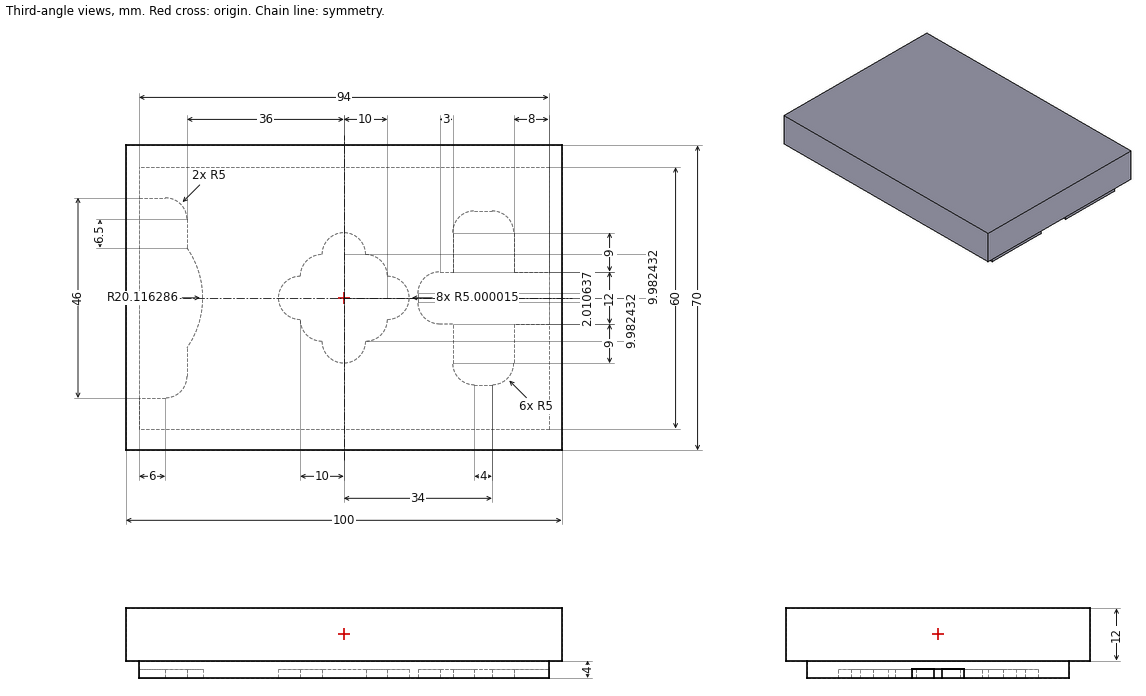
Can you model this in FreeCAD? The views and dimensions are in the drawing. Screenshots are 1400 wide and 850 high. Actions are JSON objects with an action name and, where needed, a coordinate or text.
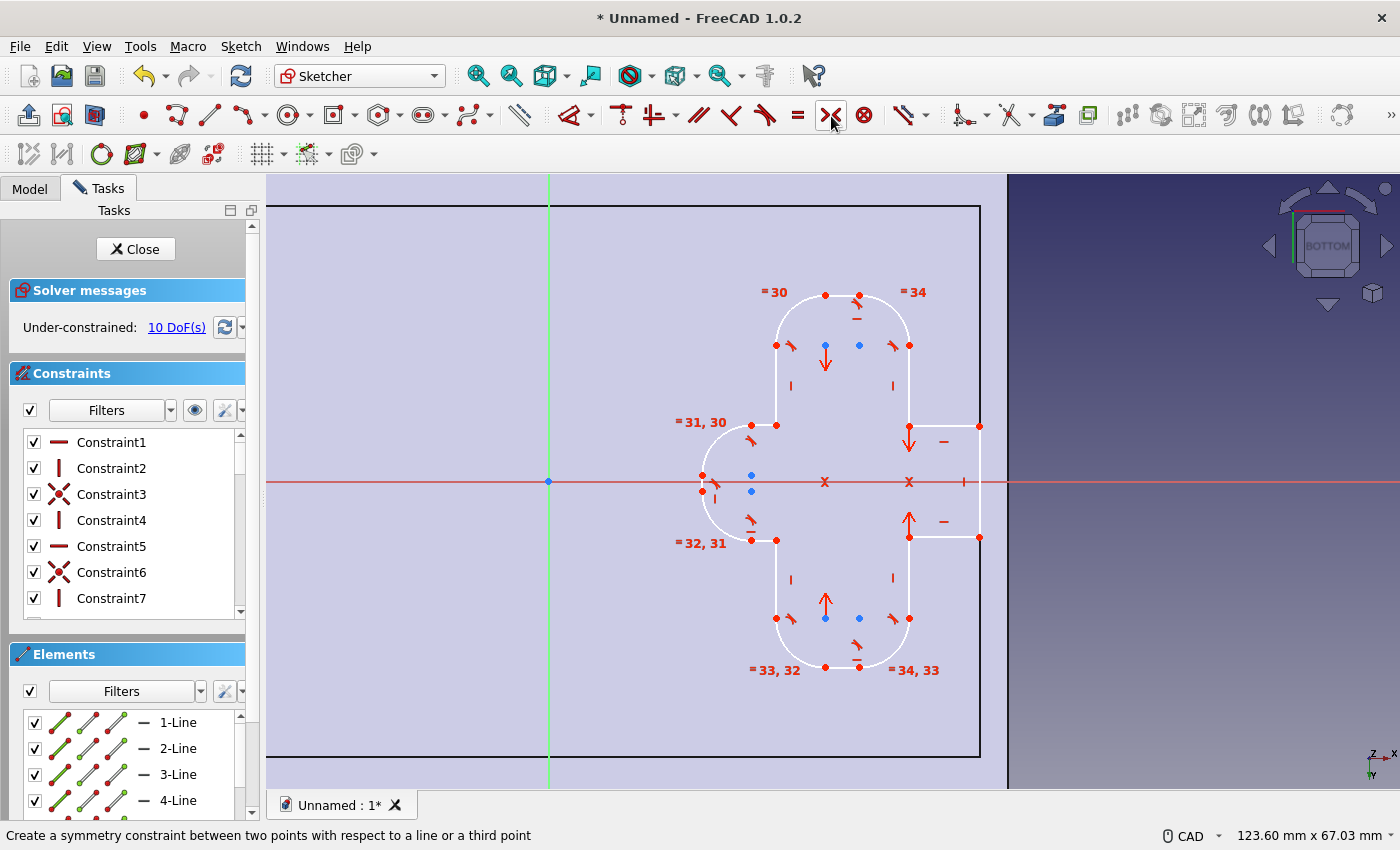
{"action": "left_click", "coordinate": [568, 116]}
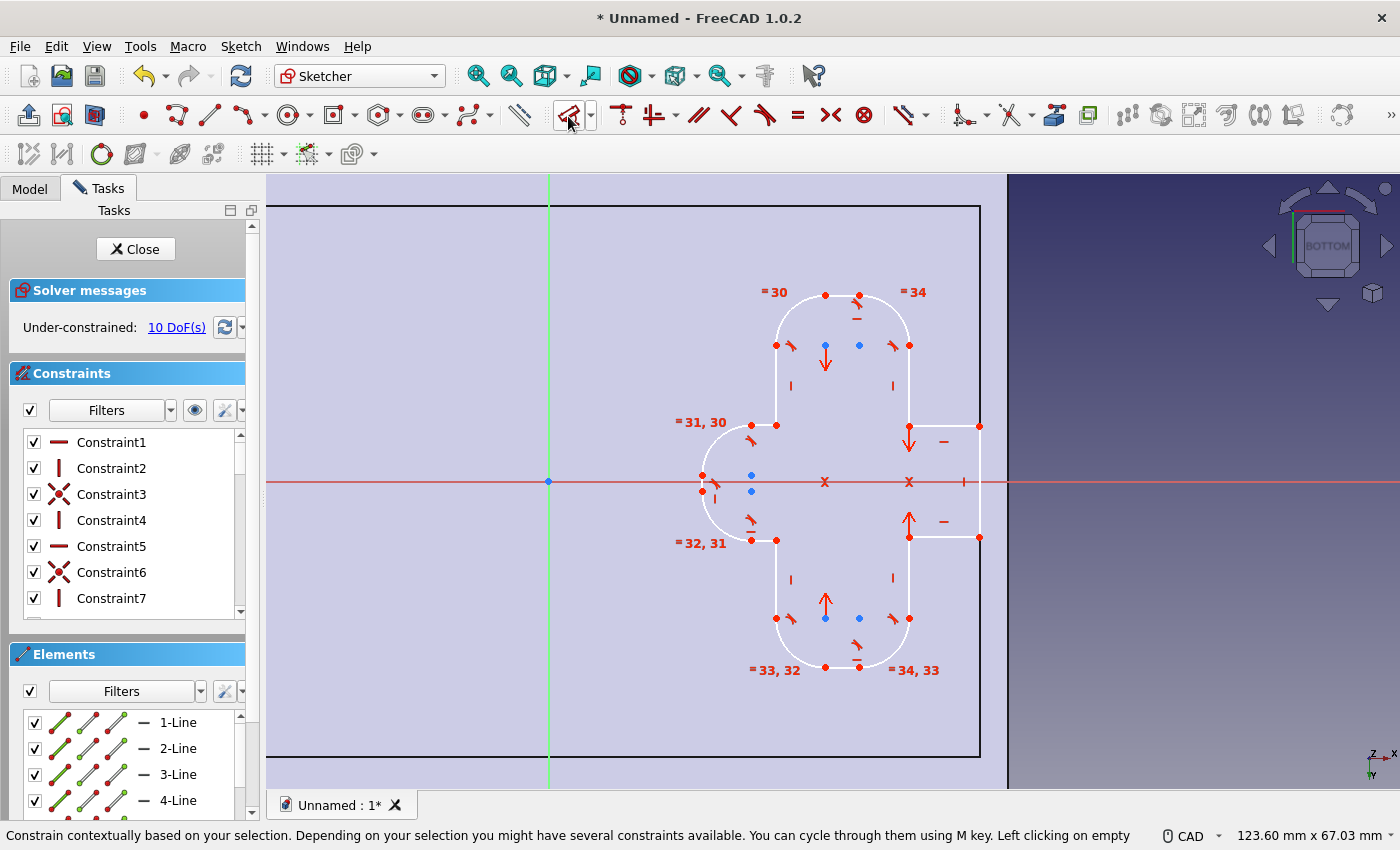
{"action": "left_click", "coordinate": [803, 301]}
{"action": "left_click", "coordinate": [788, 273]}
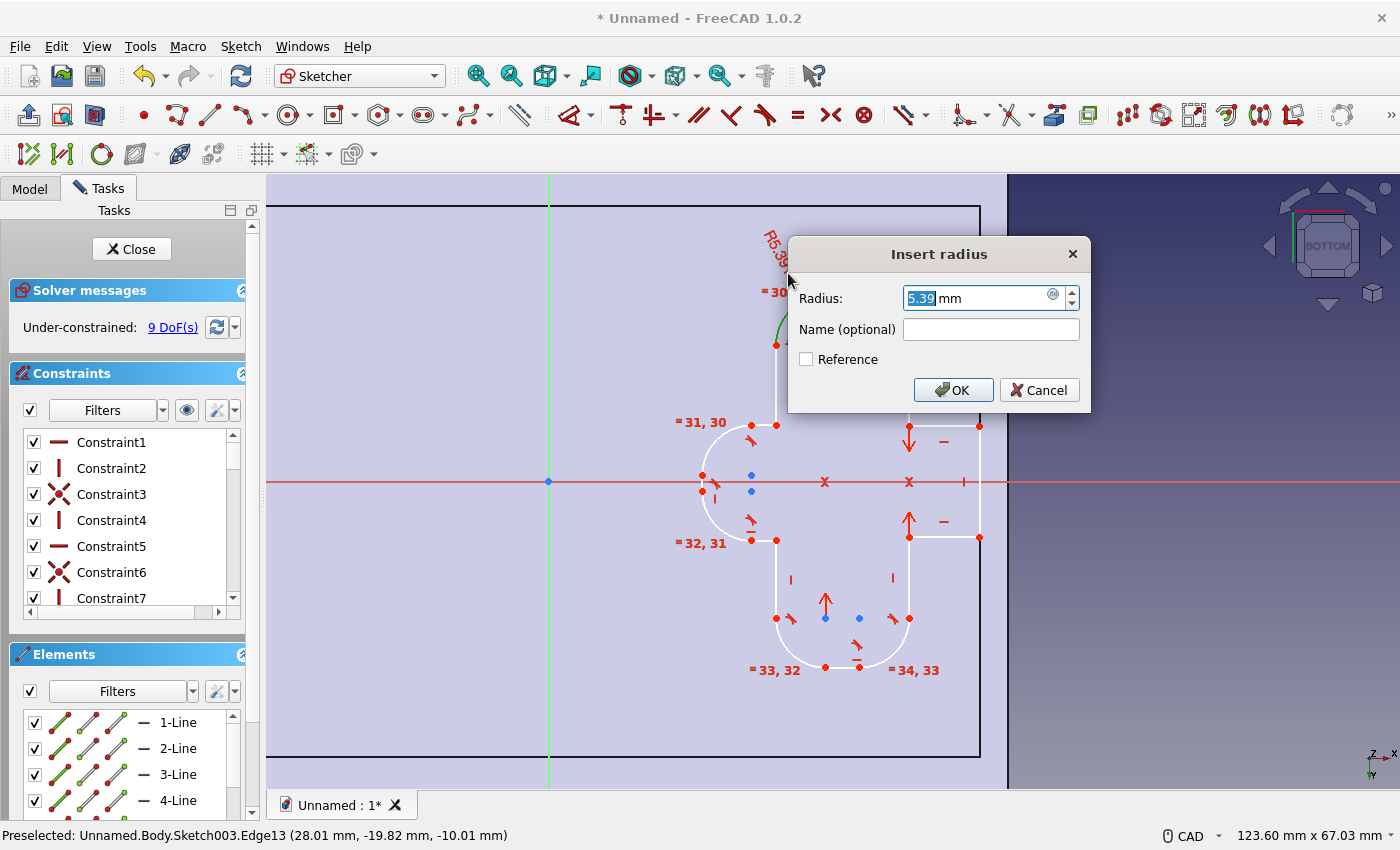
{"action": "type", "text": "5"}
{"action": "key", "text": "Return"}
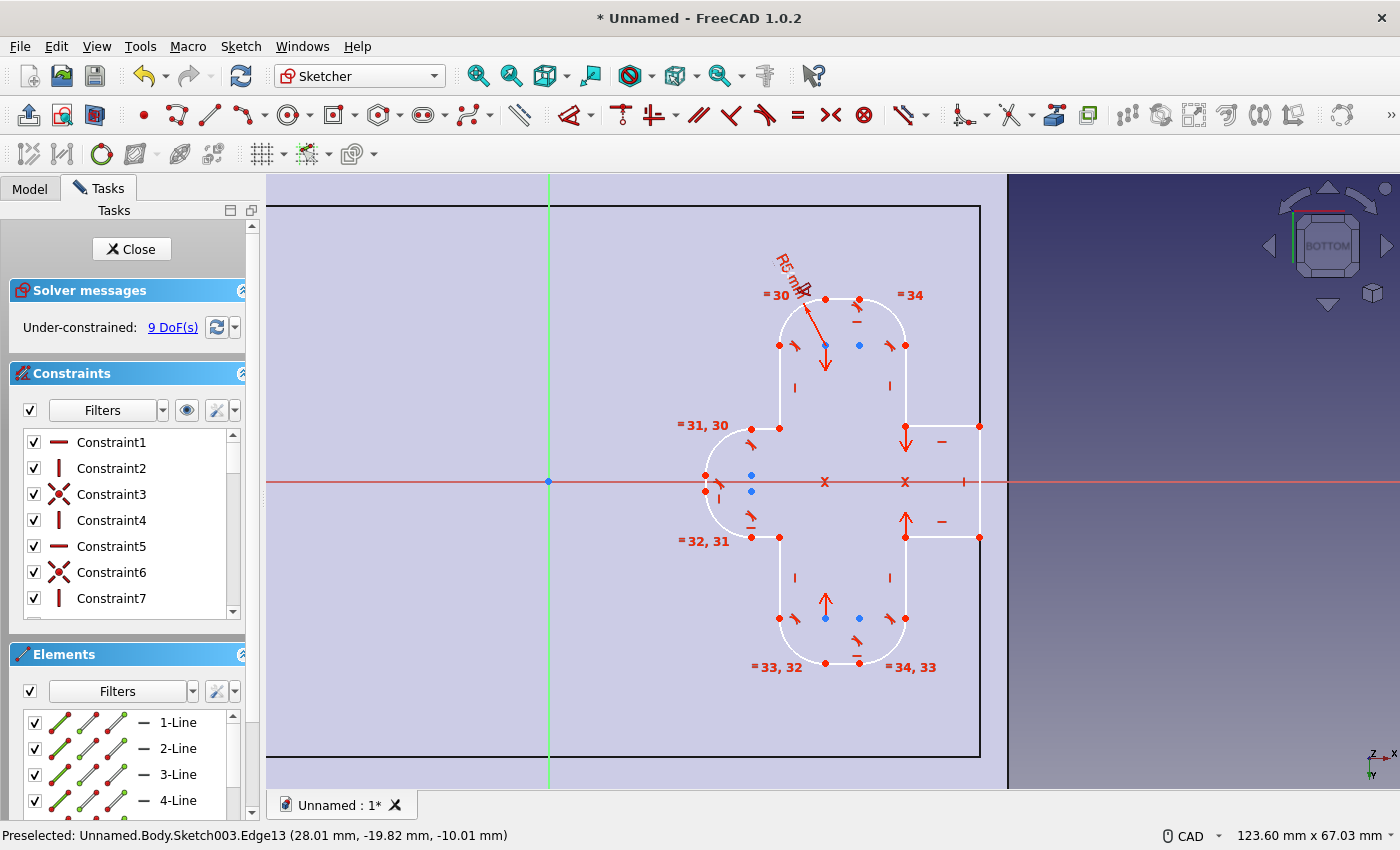
{"action": "scroll", "coordinate": [850, 299], "scroll_direction": "up", "scroll_amount": 2}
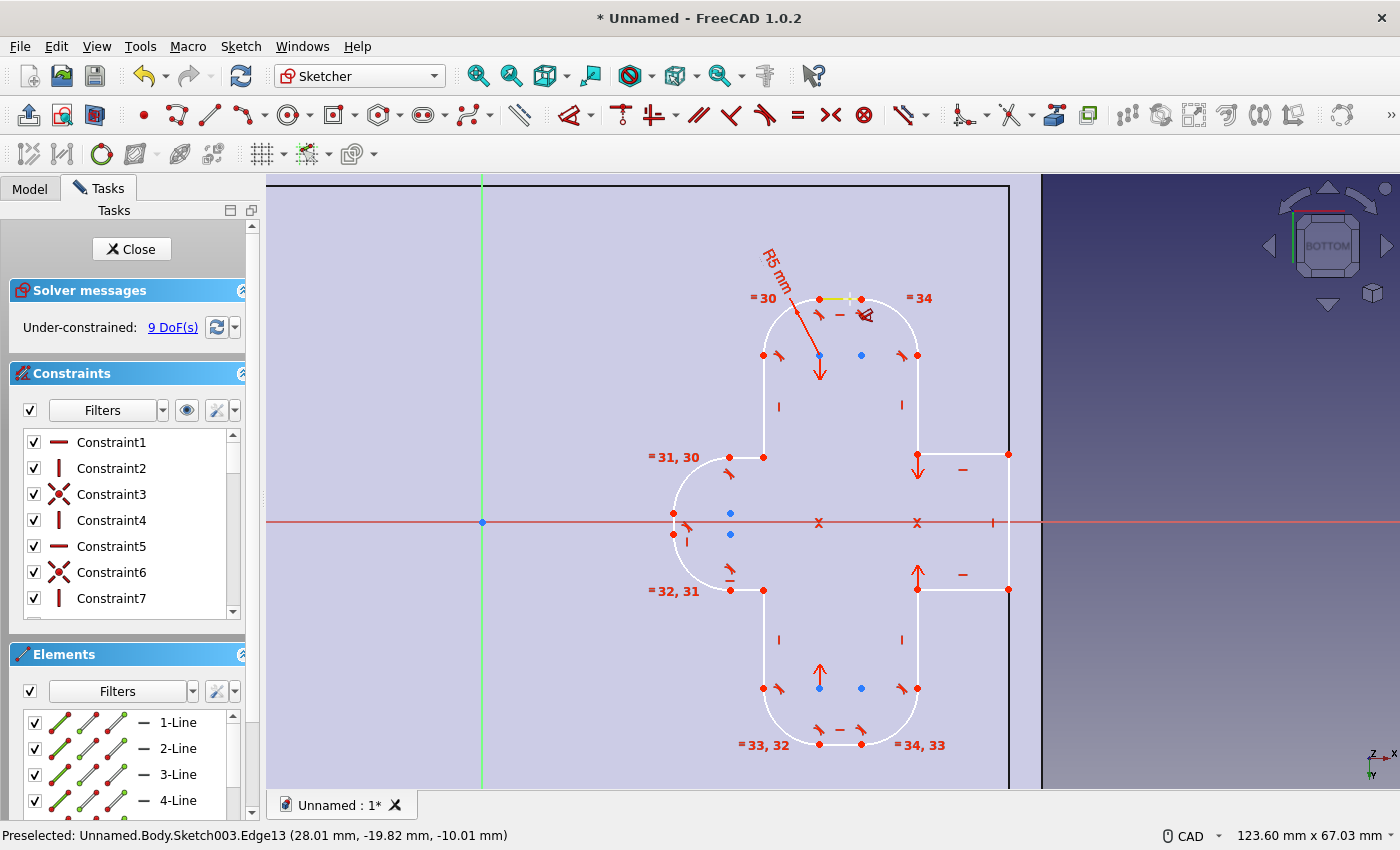
{"action": "left_click", "coordinate": [849, 299]}
{"action": "left_click", "coordinate": [839, 265]}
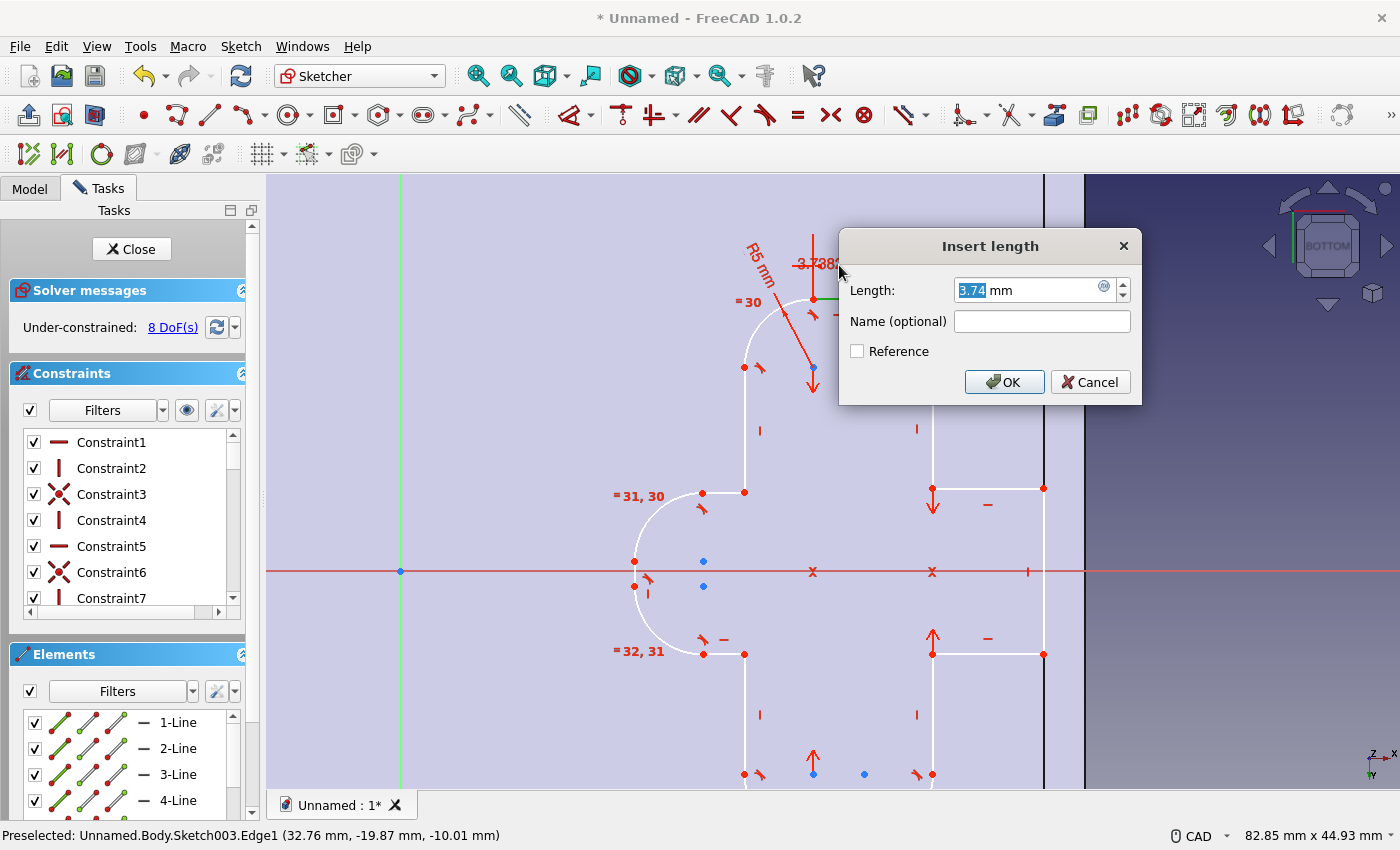
{"action": "type", "text": "4"}
{"action": "key", "text": "Return"}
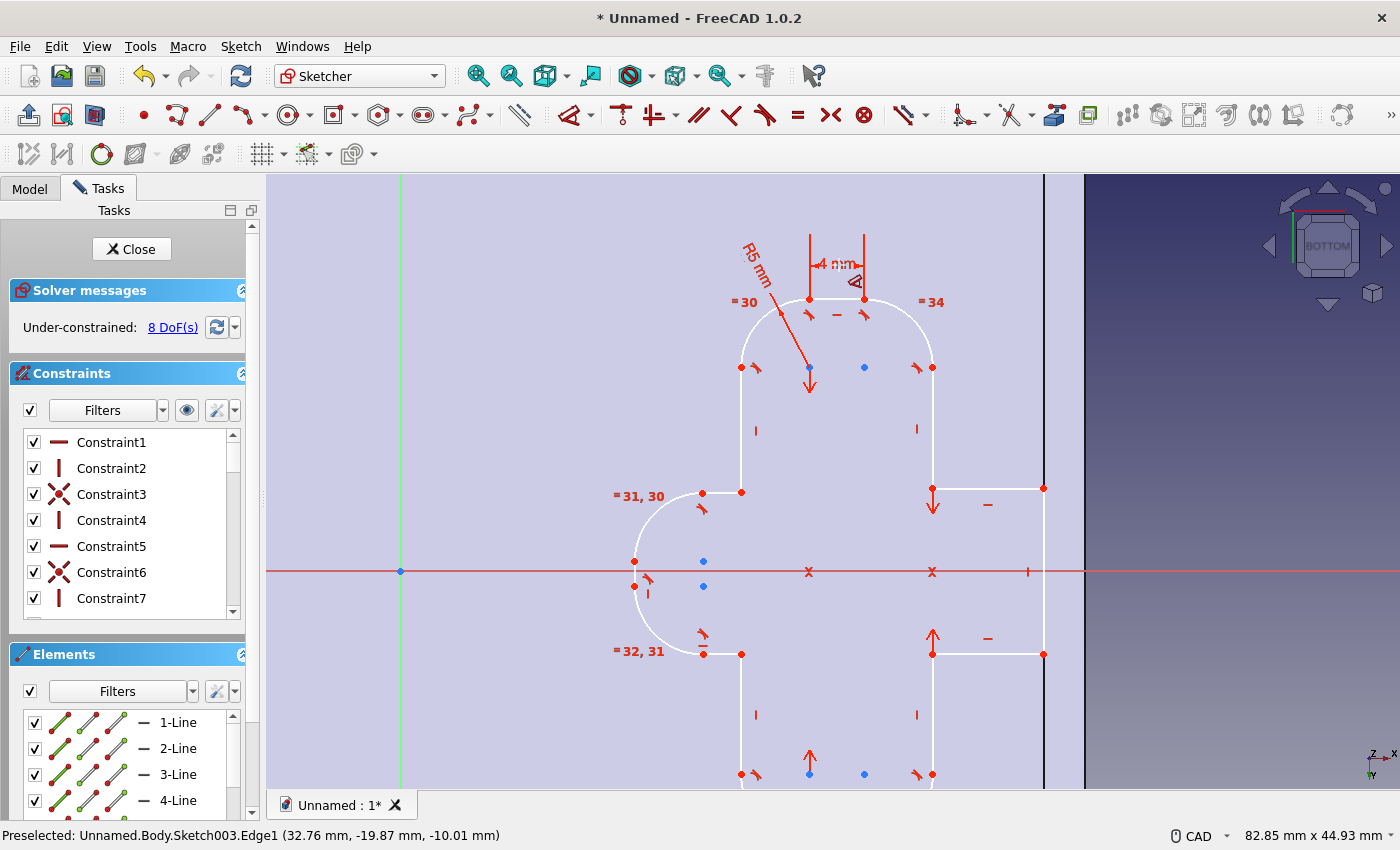
{"action": "left_click", "coordinate": [741, 405]}
{"action": "left_click", "coordinate": [775, 430]}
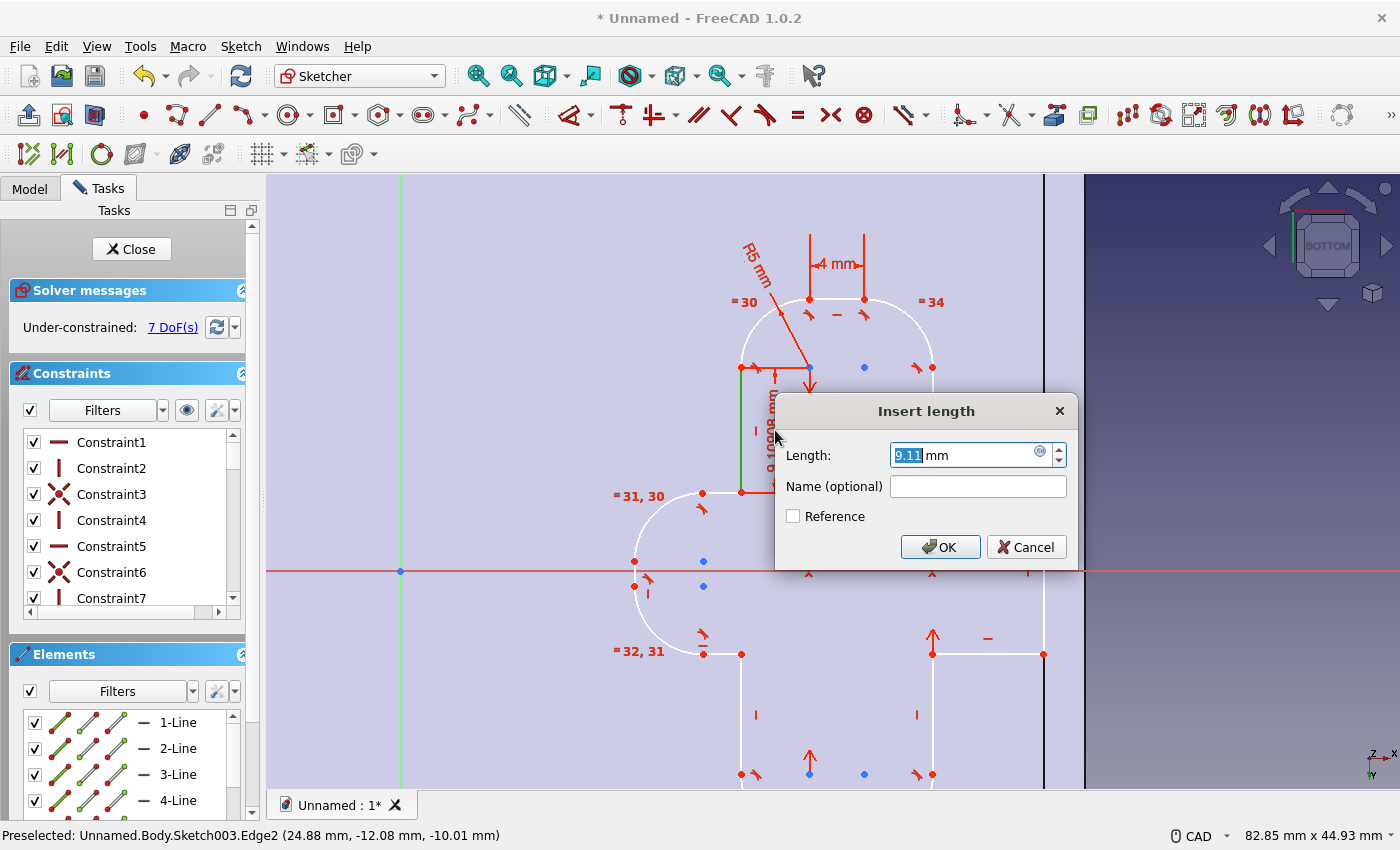
{"action": "type", "text": "9"}
{"action": "key", "text": "Return"}